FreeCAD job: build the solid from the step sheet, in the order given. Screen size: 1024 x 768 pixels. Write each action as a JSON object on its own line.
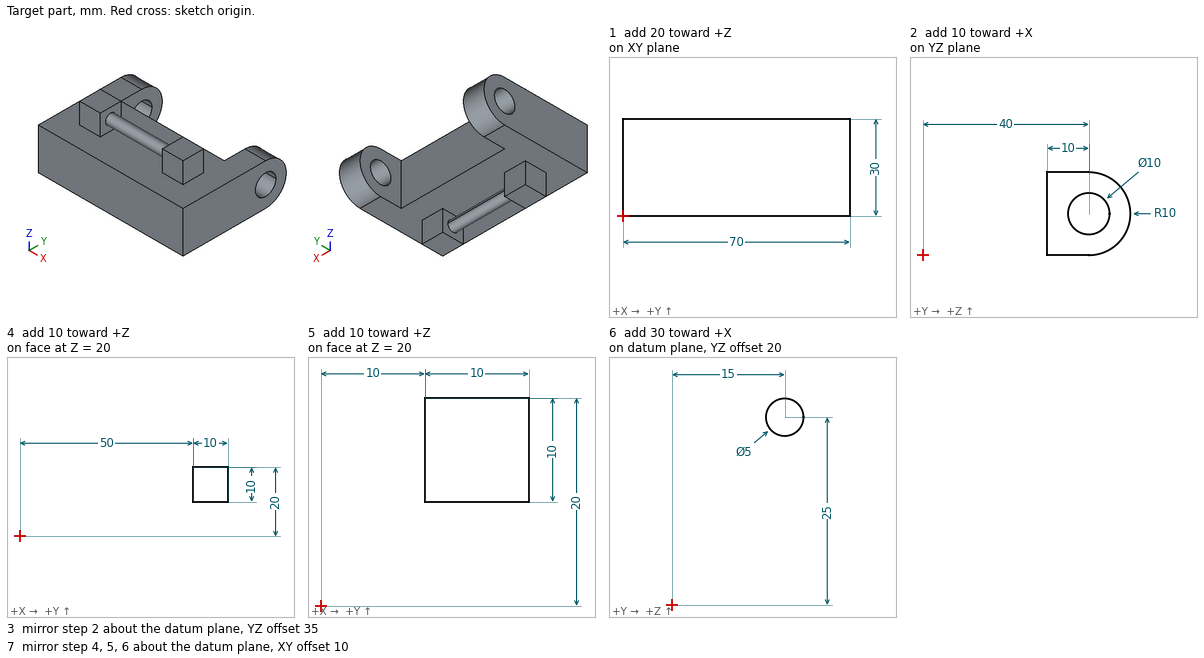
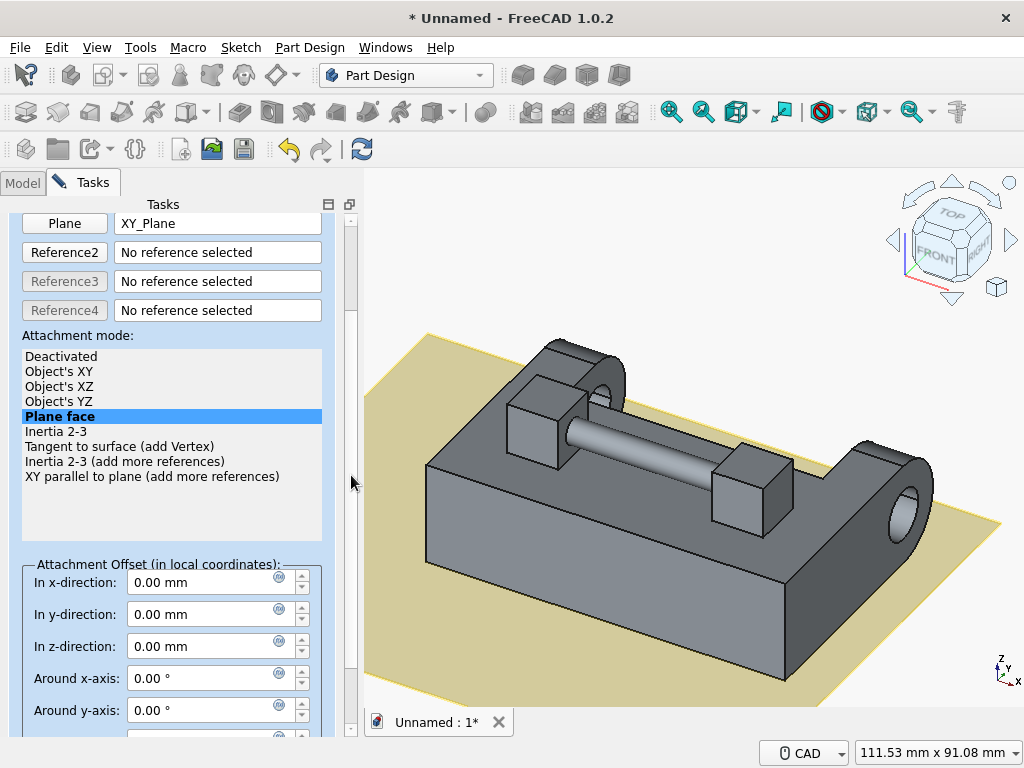
{"action": "triple_click", "coordinate": [210, 646]}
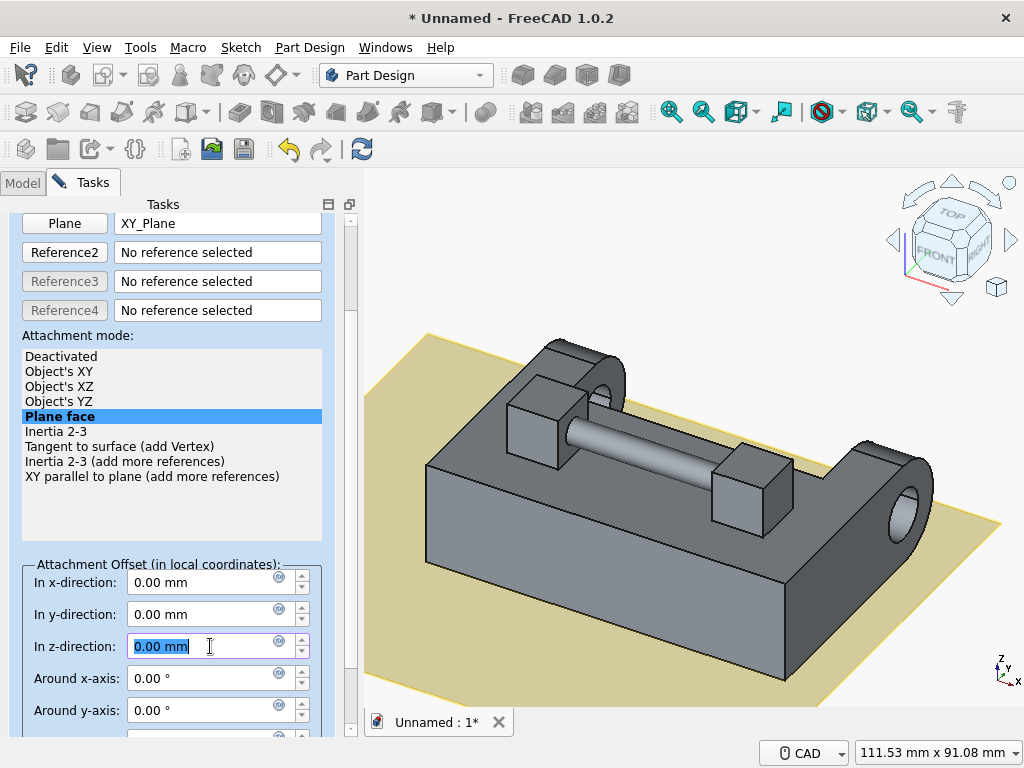
{"action": "type", "text": "10"}
{"action": "key", "text": "Tab"}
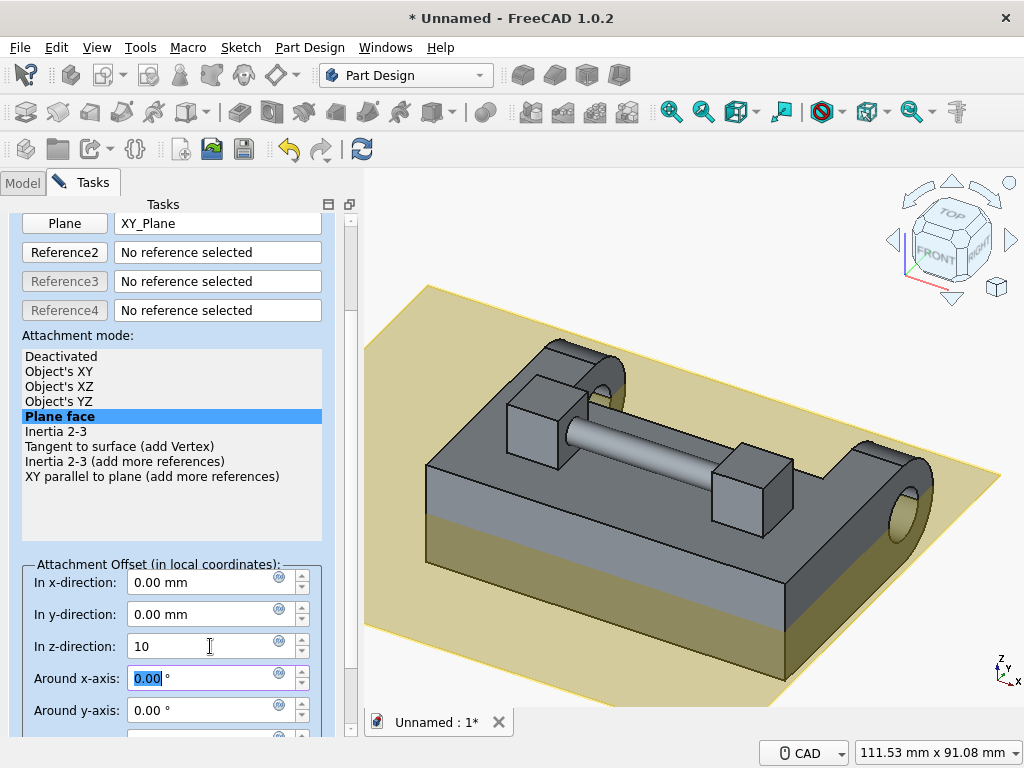
{"action": "scroll", "coordinate": [351, 475], "scroll_direction": "up", "scroll_amount": 3}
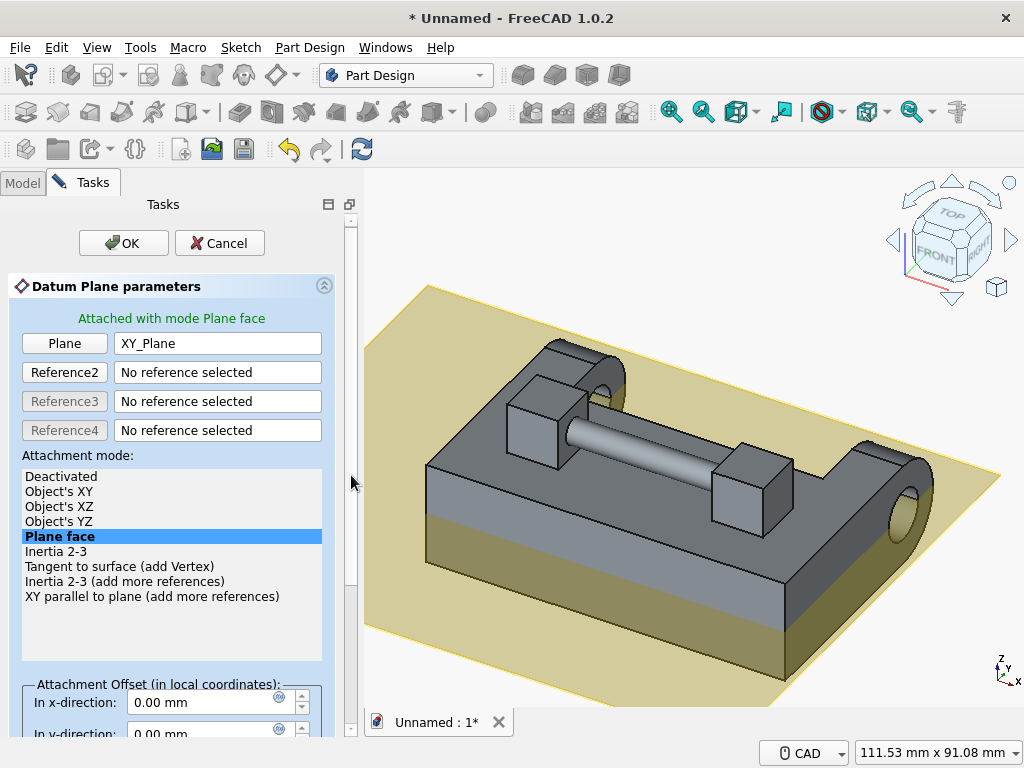
{"action": "left_click", "coordinate": [124, 243]}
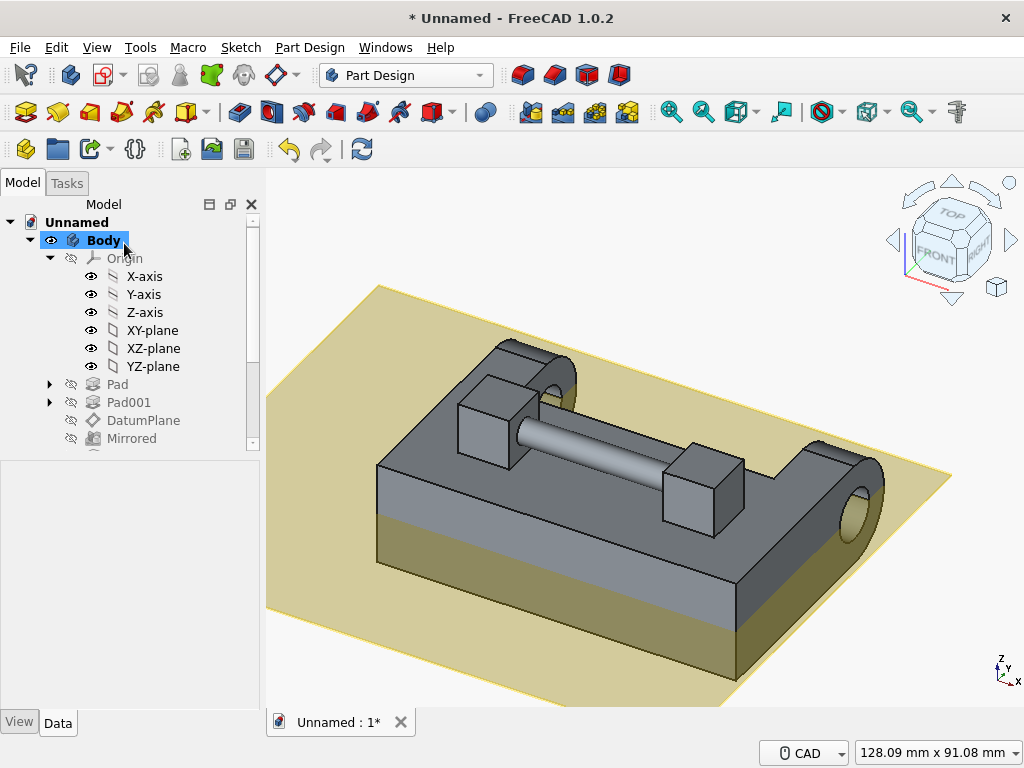
{"action": "scroll", "coordinate": [100, 326], "scroll_direction": "down", "scroll_amount": 3}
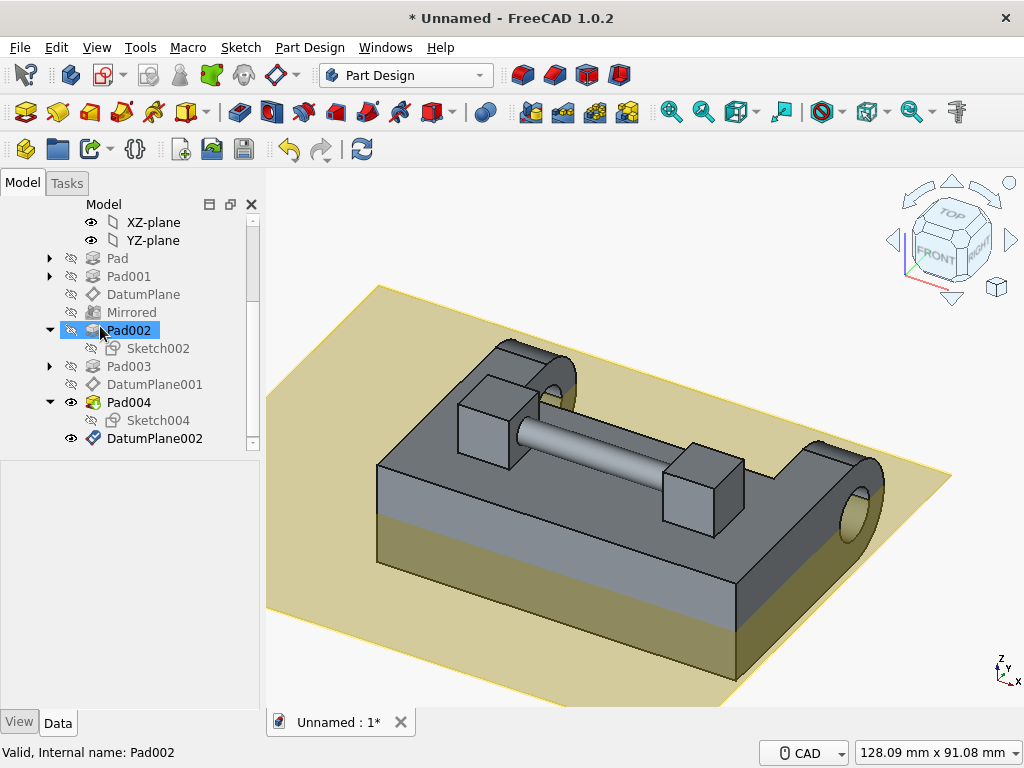
{"action": "left_click", "coordinate": [116, 330]}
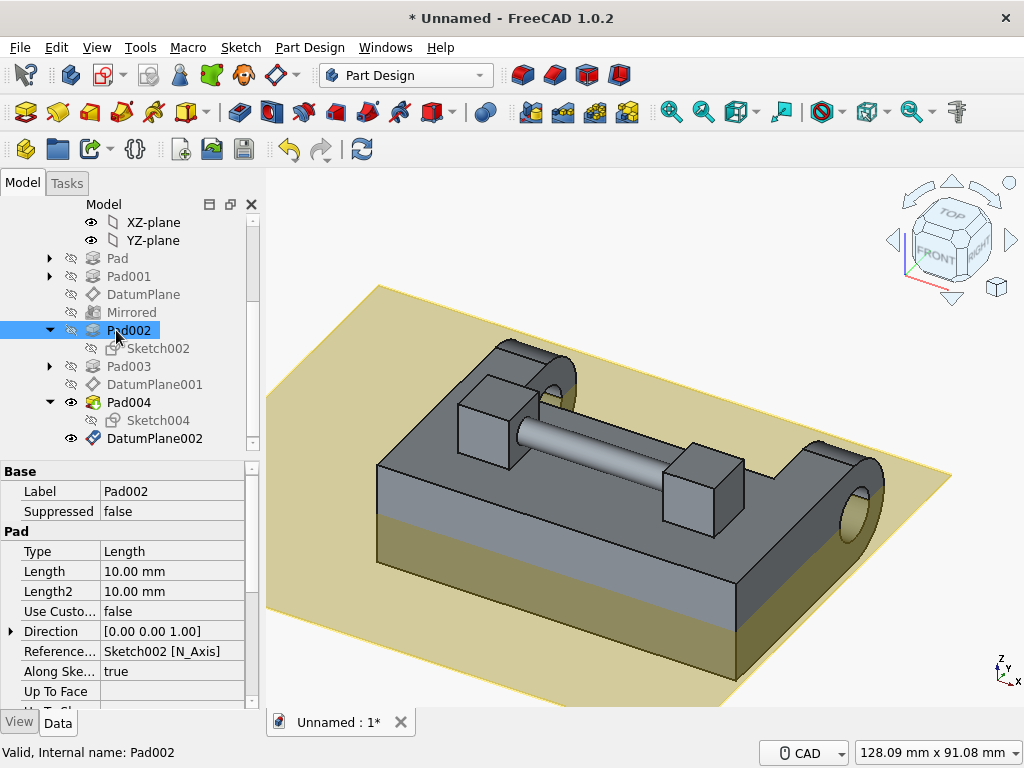
{"action": "left_click", "coordinate": [116, 366], "text": "ctrl"}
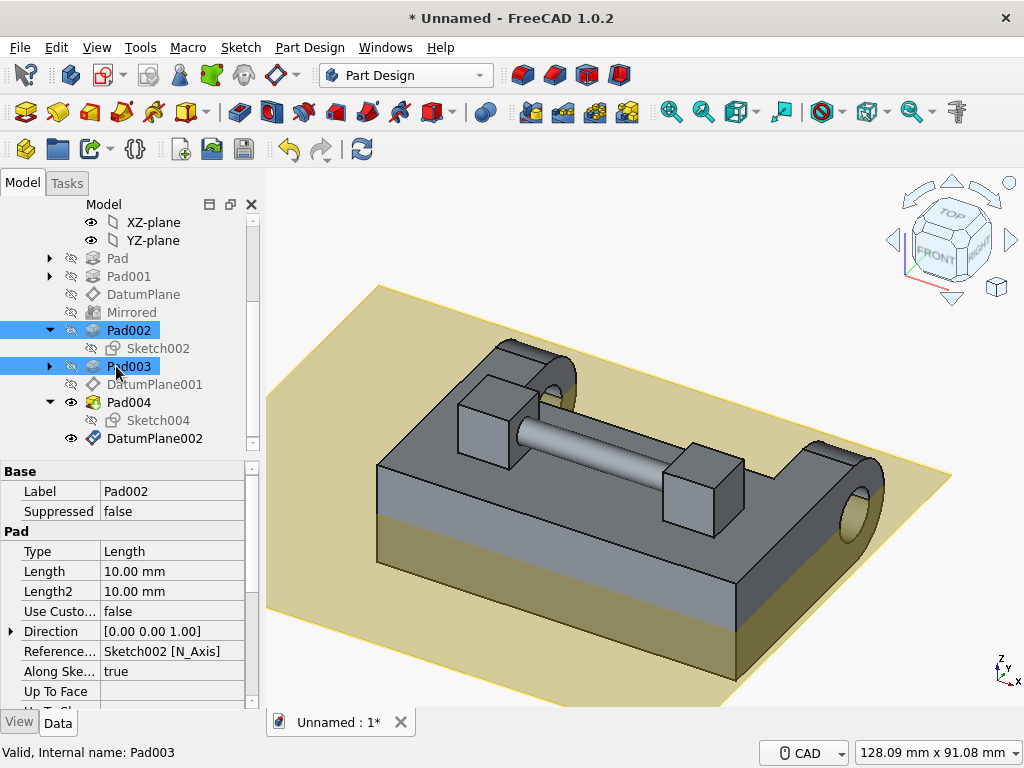
{"action": "left_click", "coordinate": [116, 402], "text": "ctrl"}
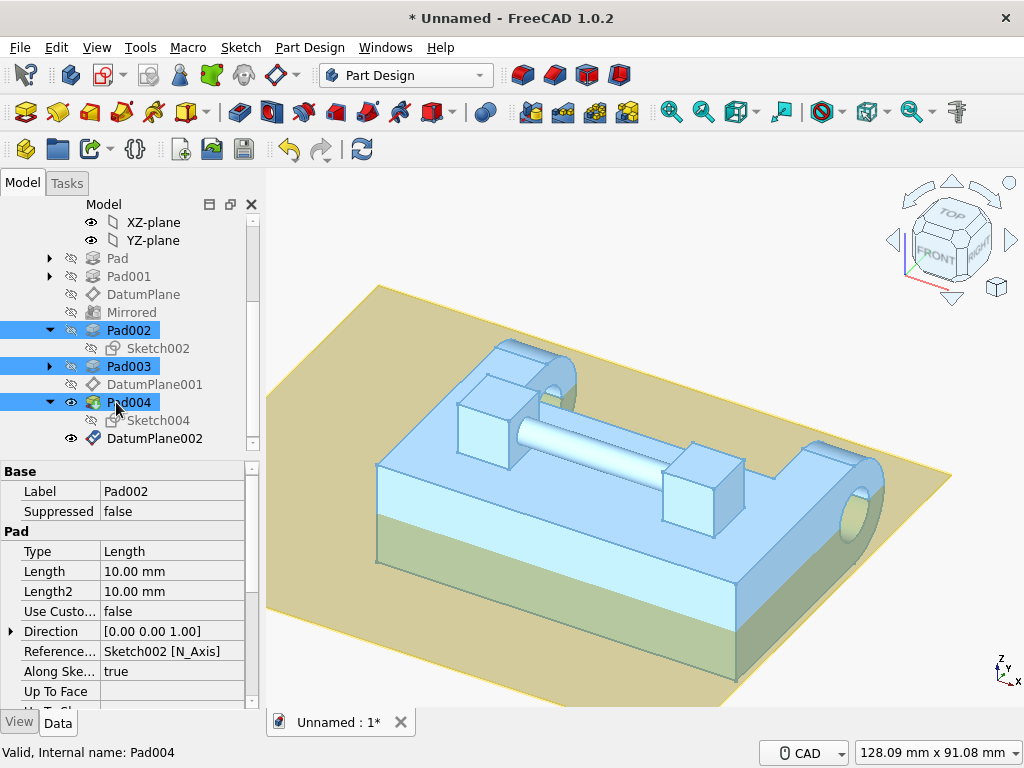
{"action": "left_click", "coordinate": [532, 112]}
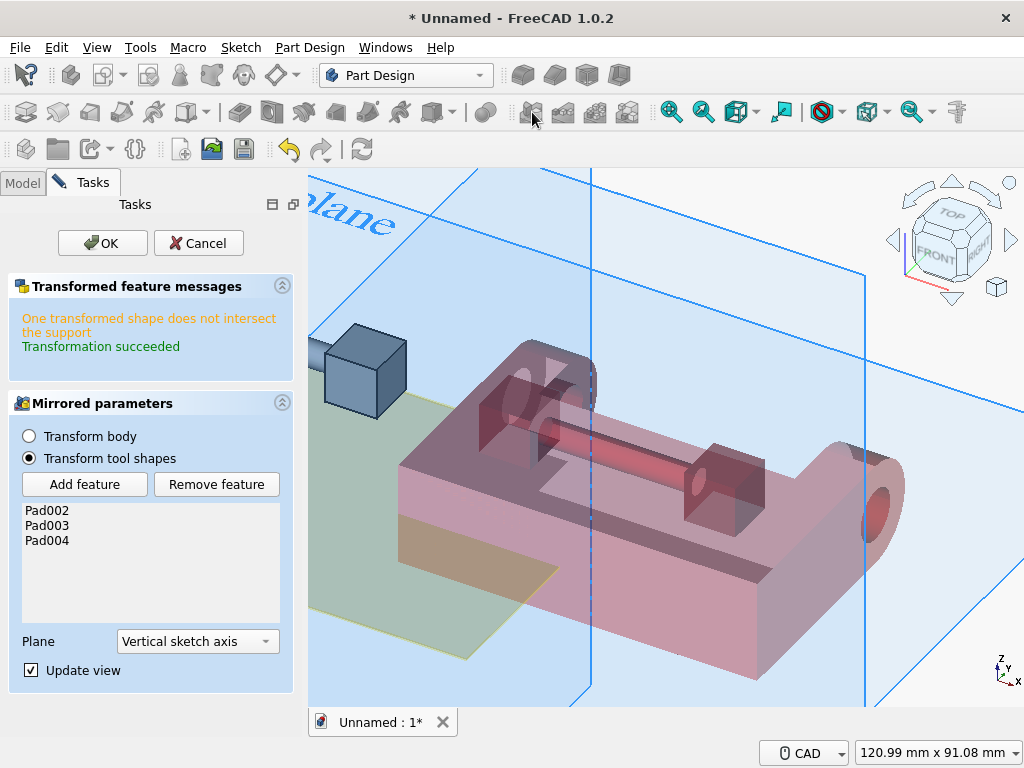
{"action": "left_click", "coordinate": [198, 642]}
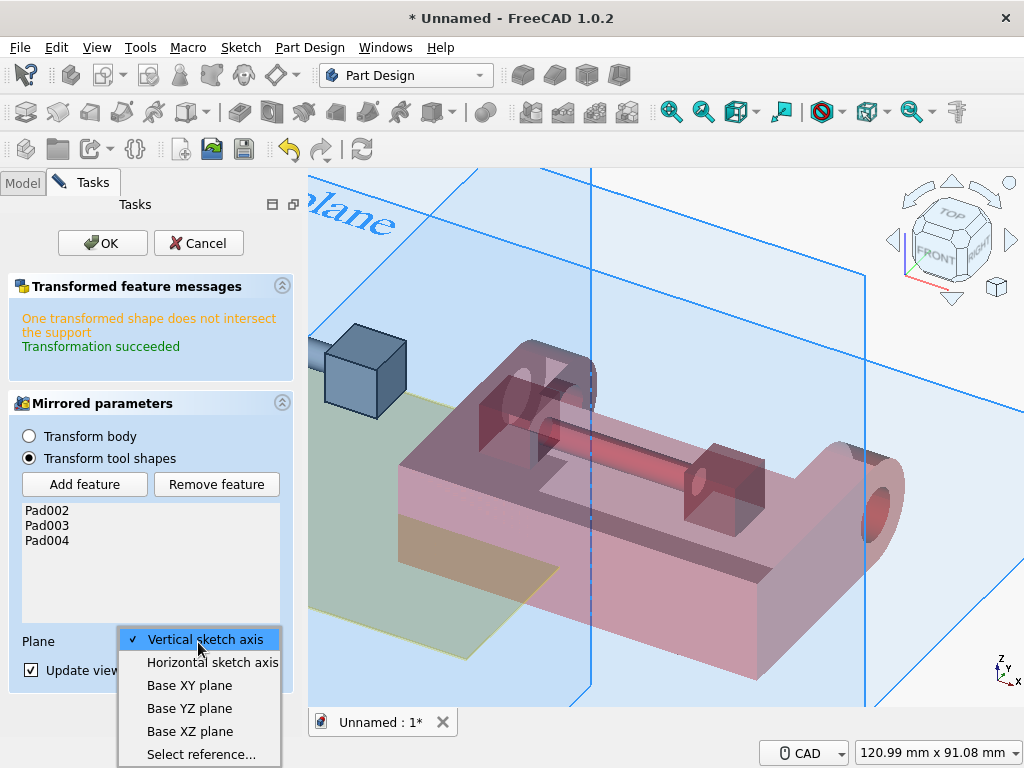
{"action": "left_click", "coordinate": [198, 754]}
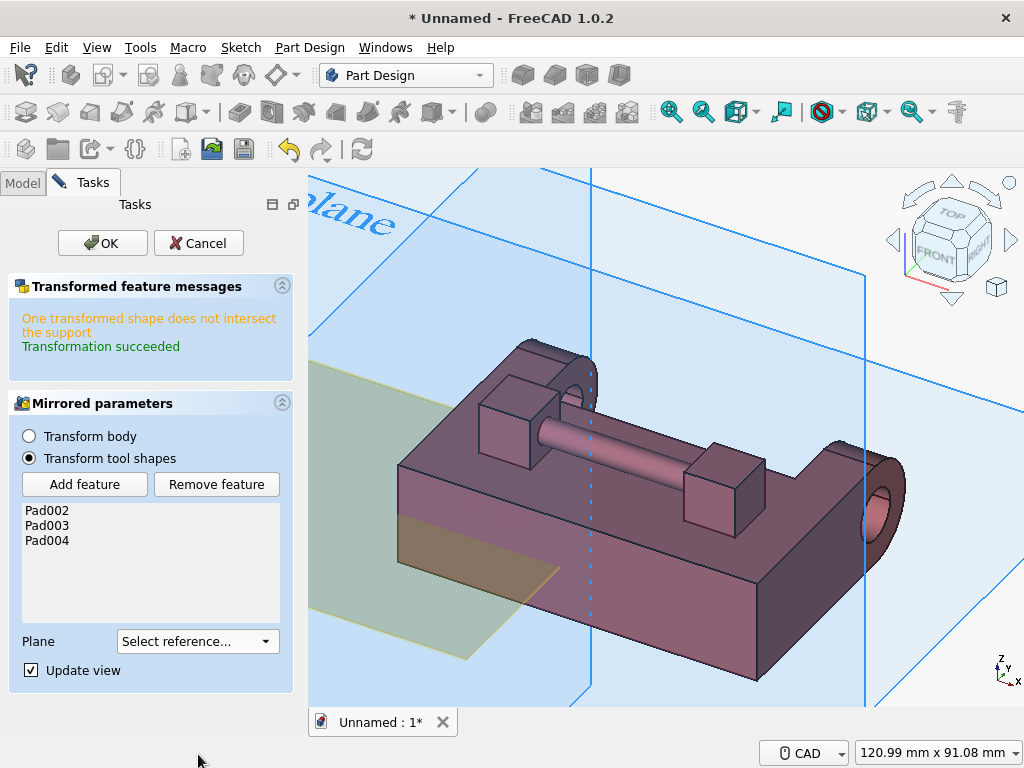
{"action": "left_click", "coordinate": [23, 182]}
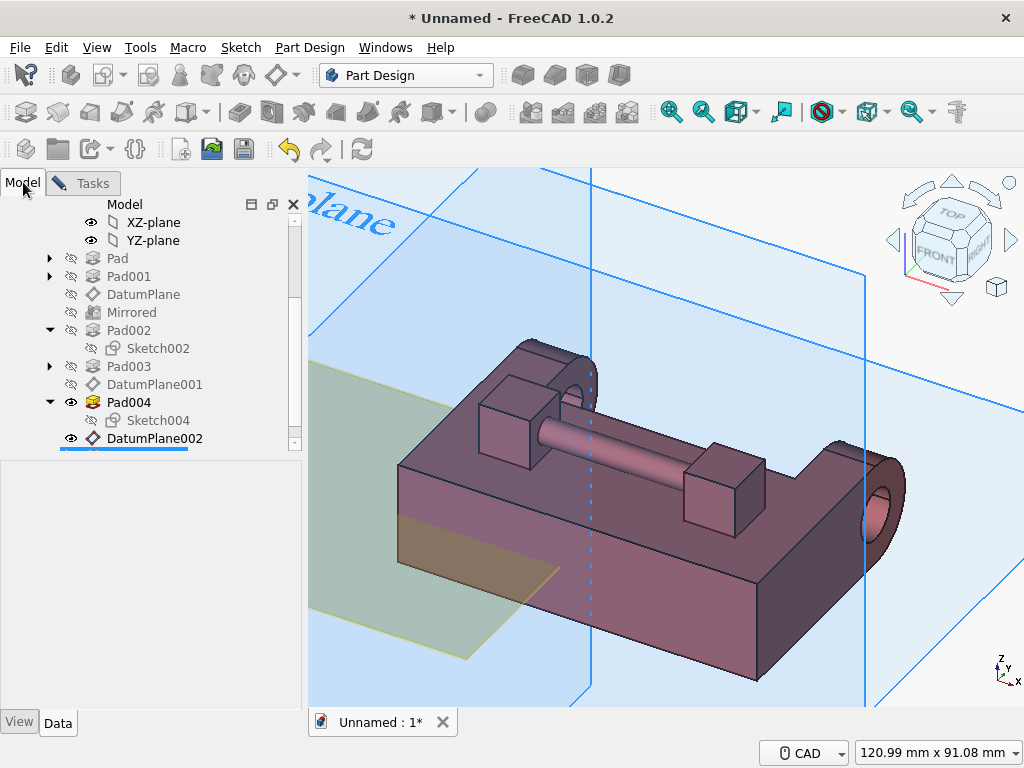
{"action": "left_click", "coordinate": [116, 438]}